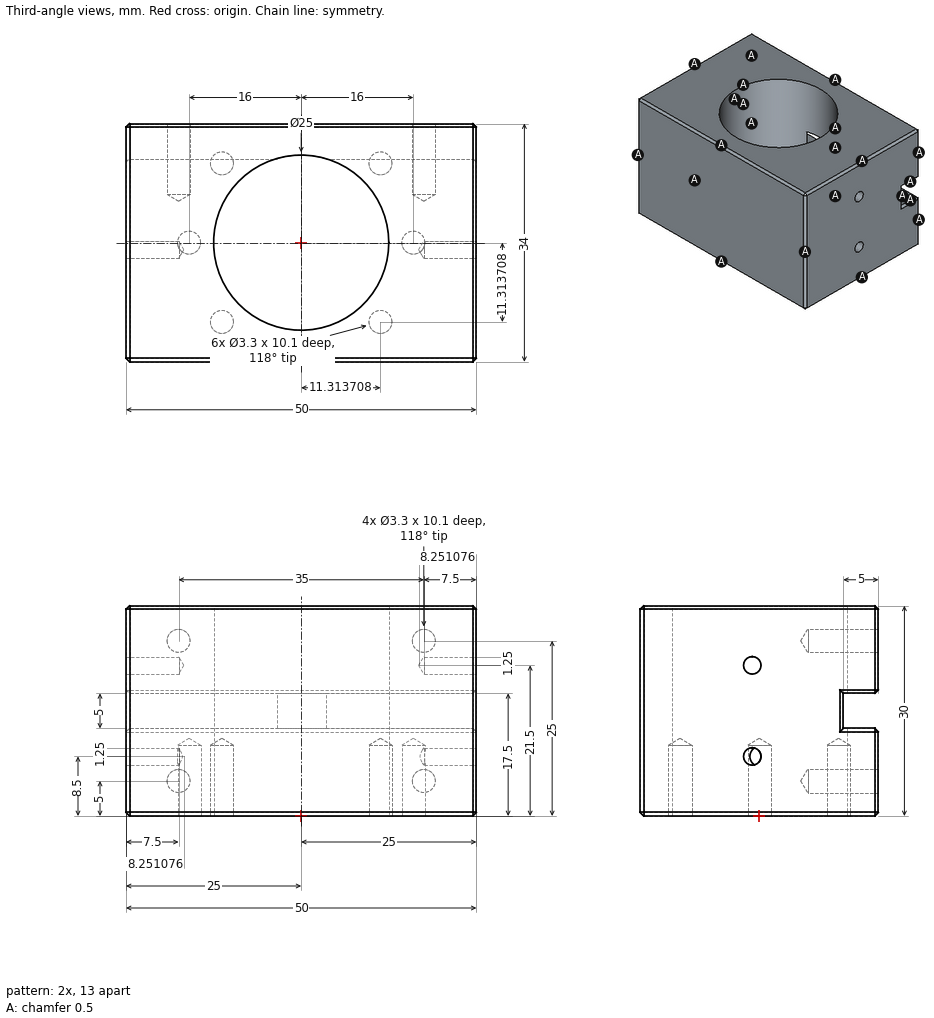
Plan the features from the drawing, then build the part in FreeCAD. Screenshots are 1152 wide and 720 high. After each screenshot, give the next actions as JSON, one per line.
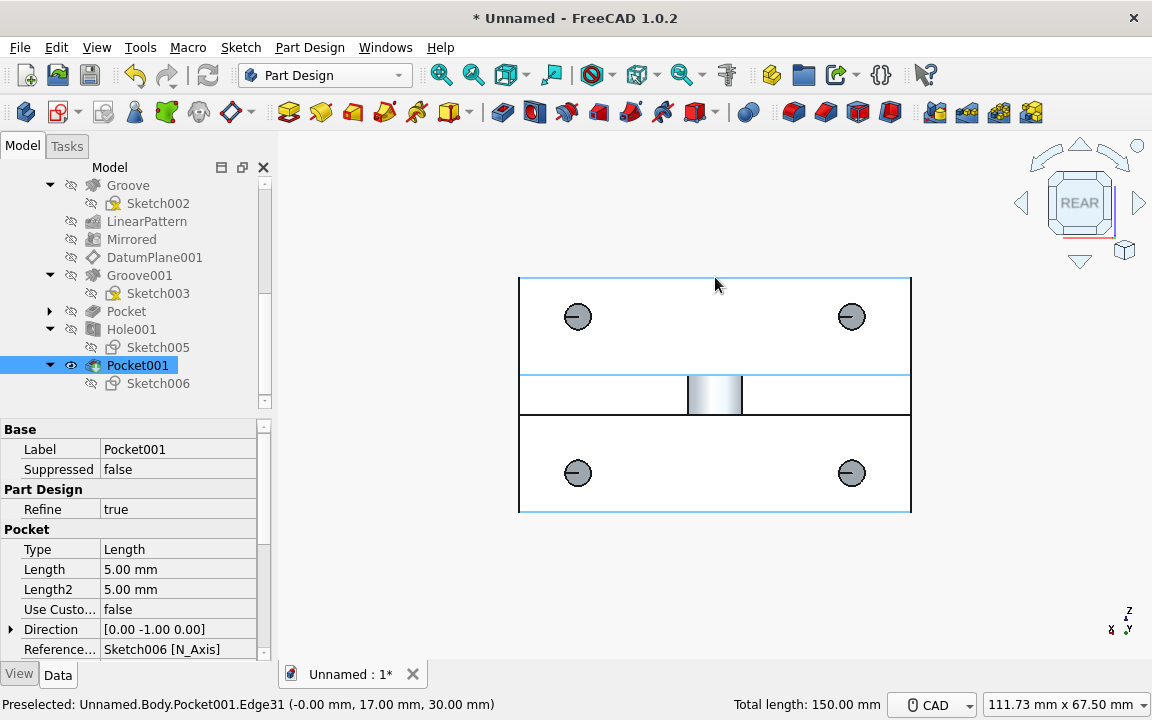
{"action": "left_click", "coordinate": [911, 326], "text": "ctrl"}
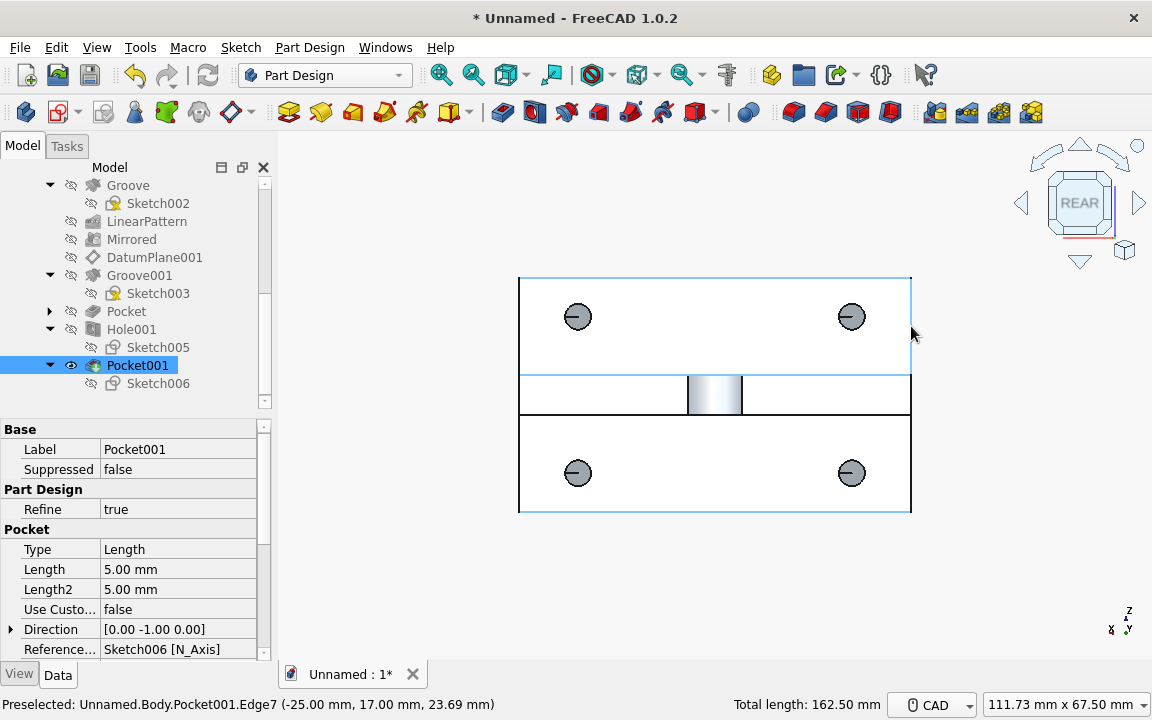
{"action": "left_click", "coordinate": [911, 462], "text": "ctrl"}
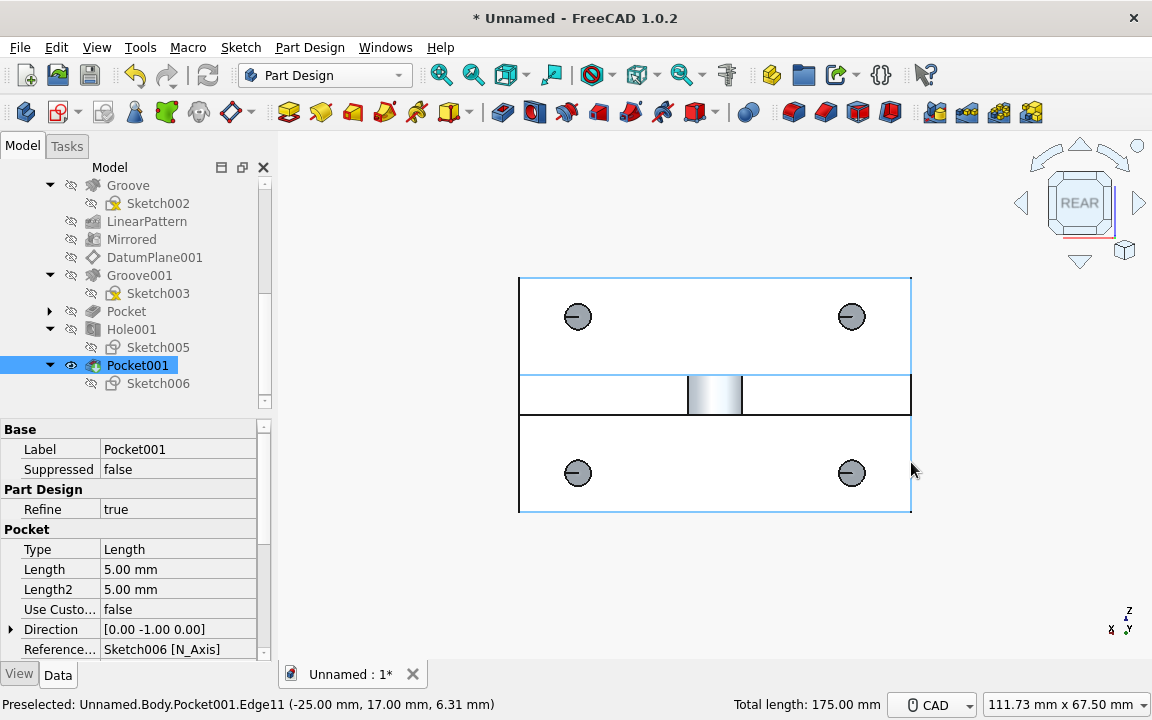
{"action": "left_click", "coordinate": [911, 394], "text": "ctrl"}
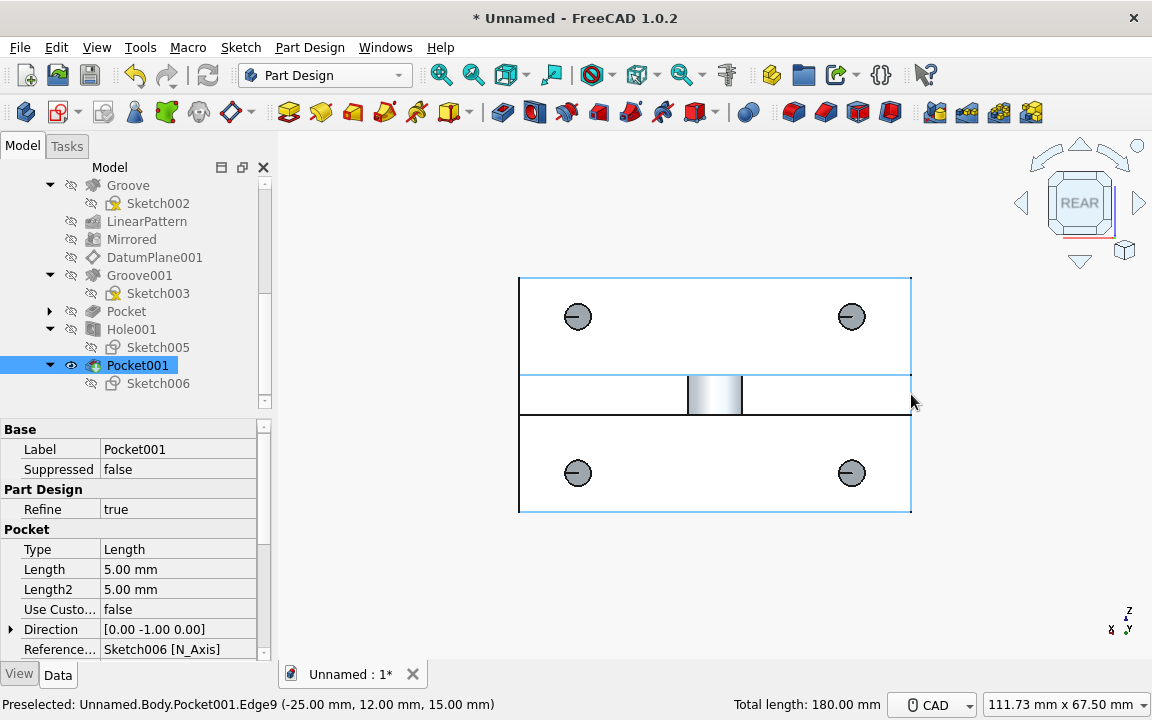
{"action": "left_click", "coordinate": [715, 414], "text": "ctrl"}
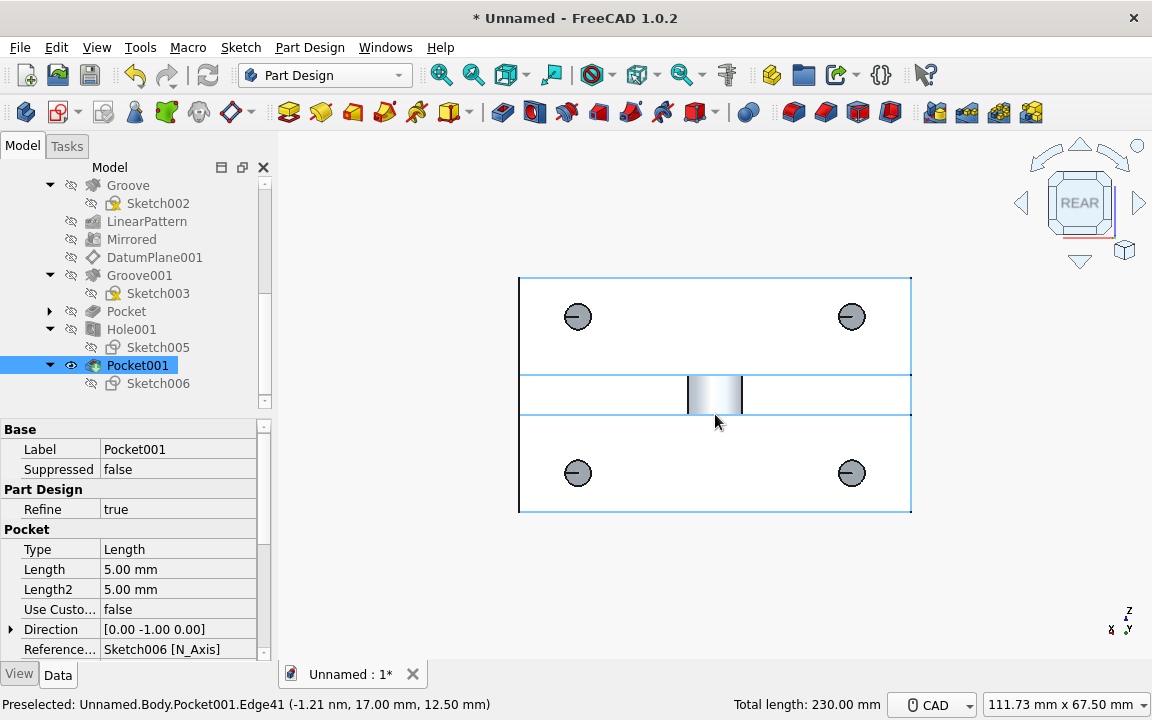
{"action": "key", "text": "0"}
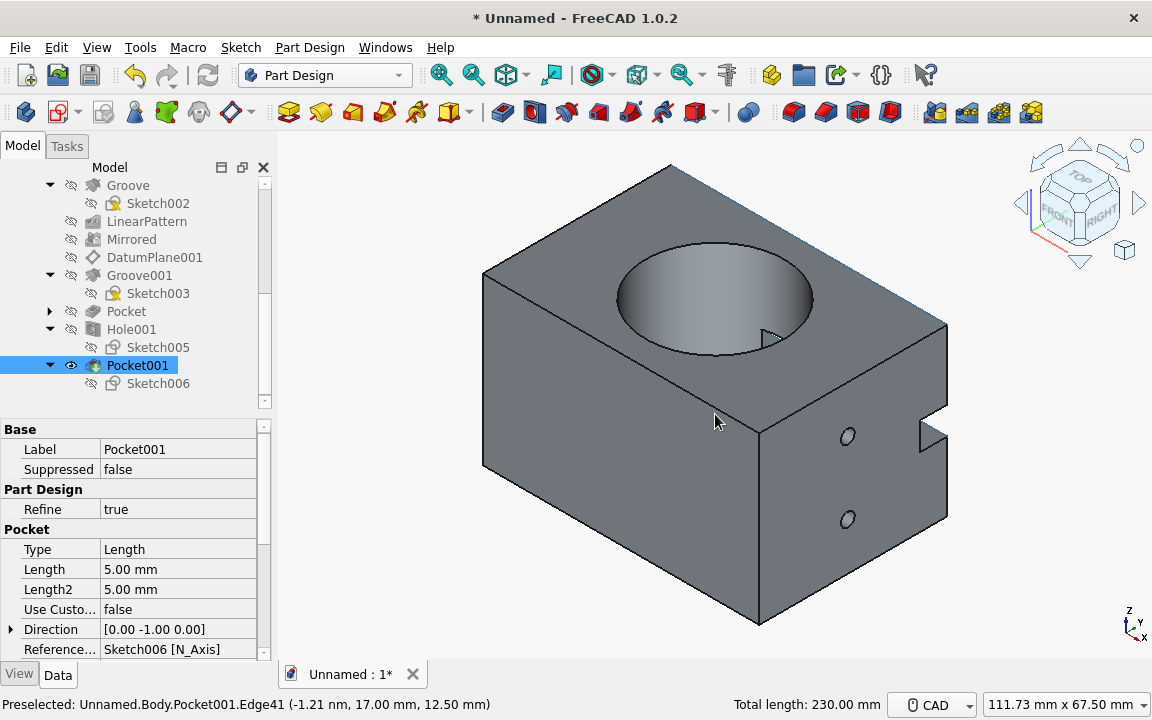
{"action": "left_click", "coordinate": [660, 471], "text": "ctrl"}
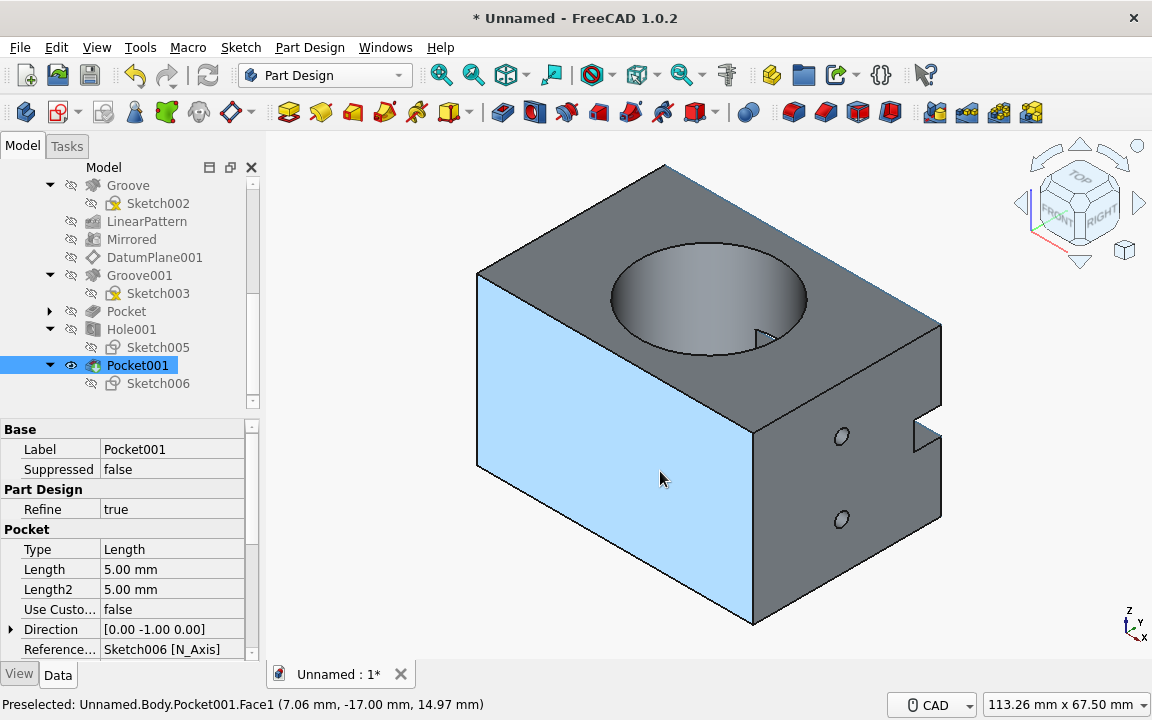
{"action": "left_click", "coordinate": [847, 378], "text": "ctrl"}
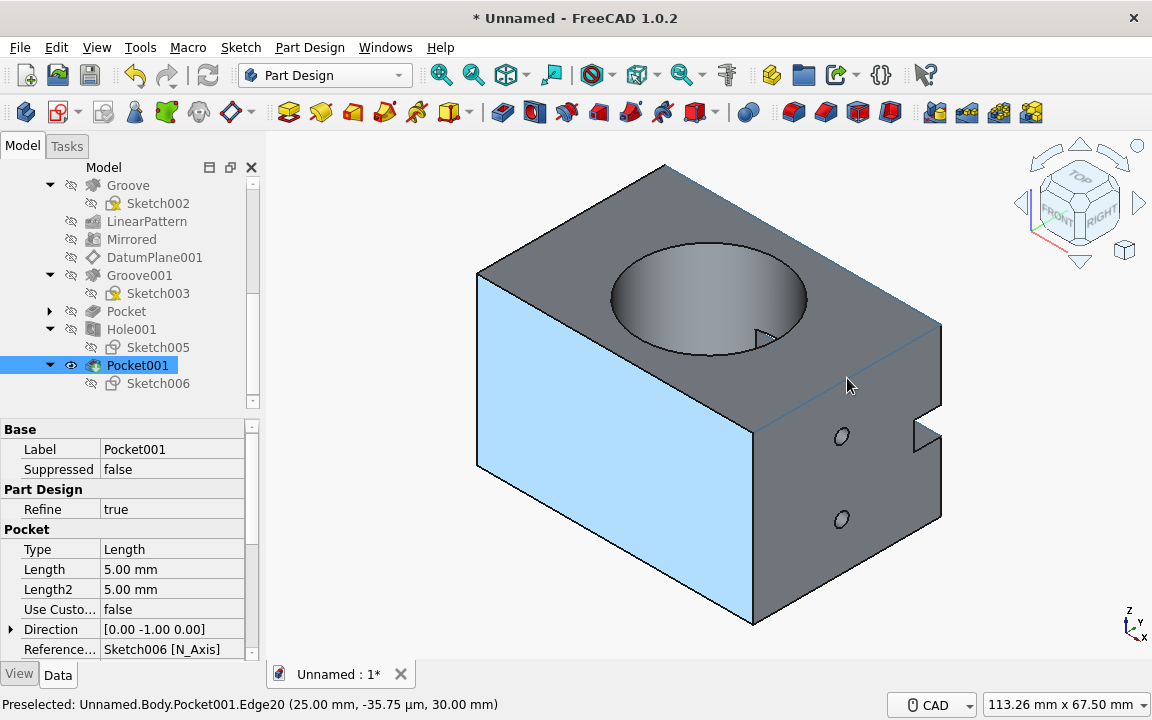
{"action": "left_click", "coordinate": [927, 443], "text": "ctrl"}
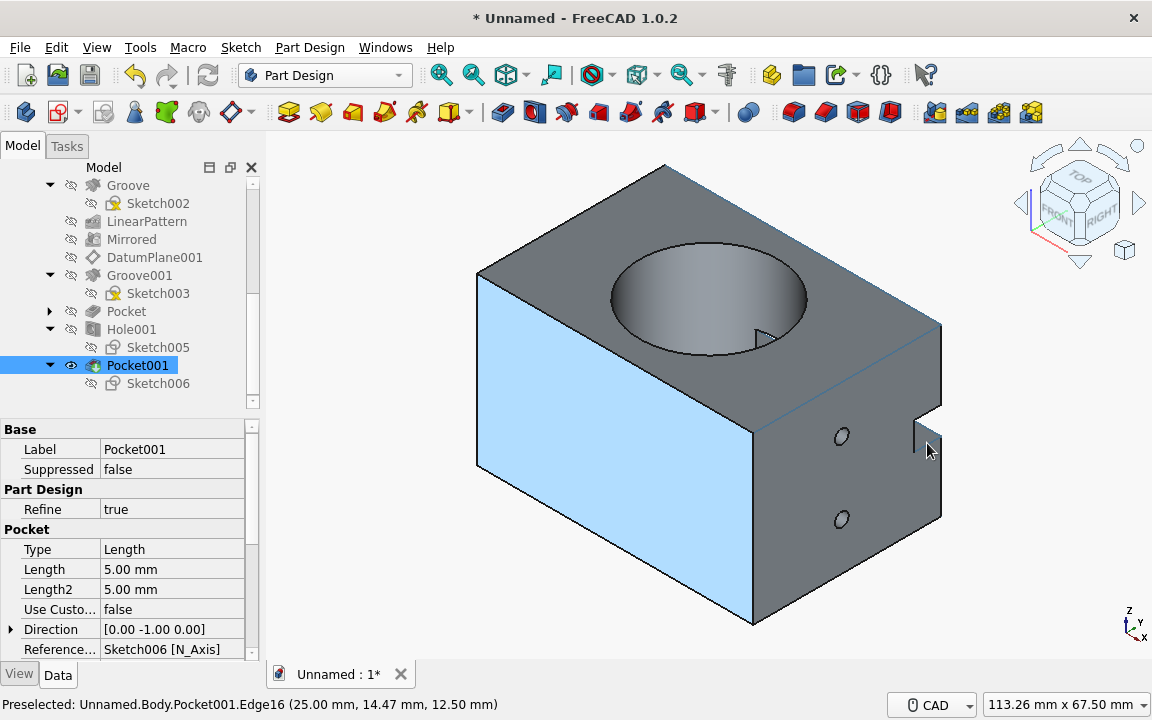
{"action": "key", "text": "2"}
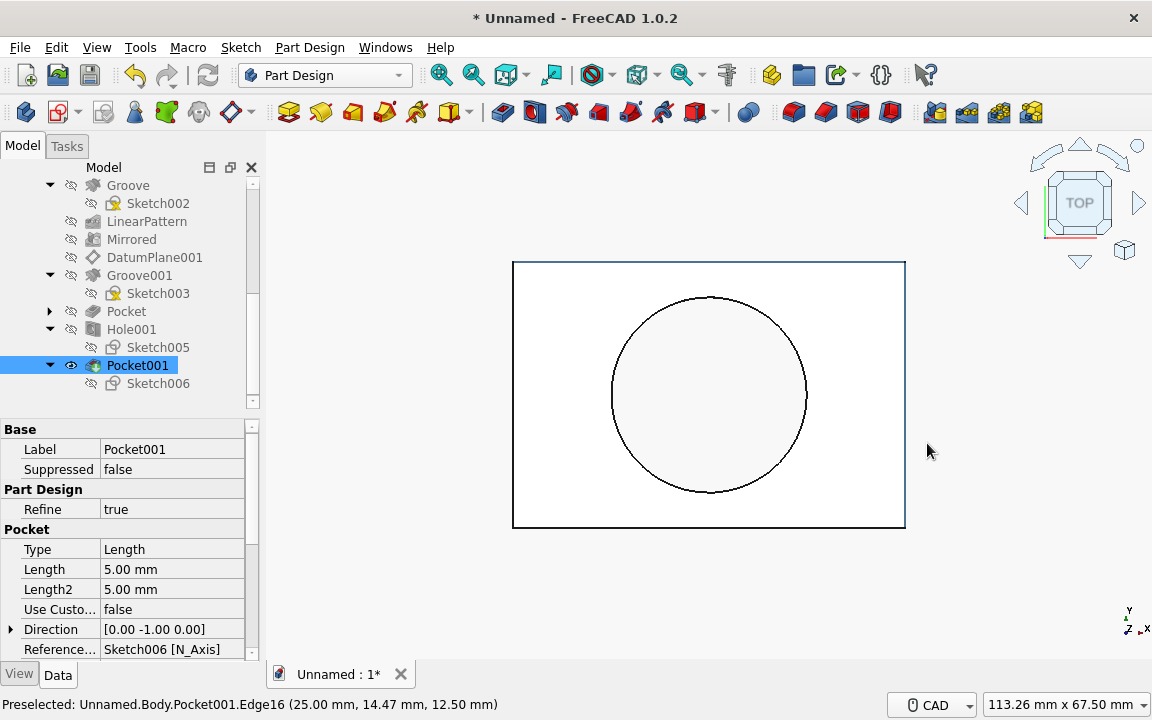
{"action": "left_click", "coordinate": [513, 394], "text": "ctrl"}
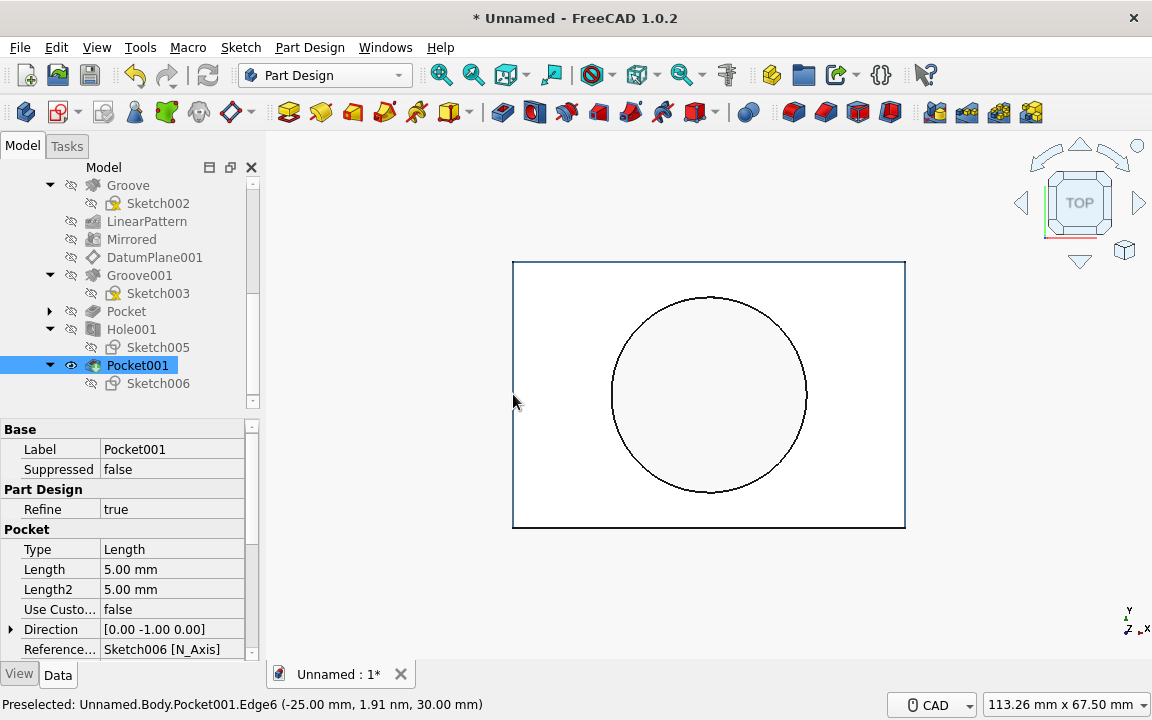
{"action": "key", "text": "1"}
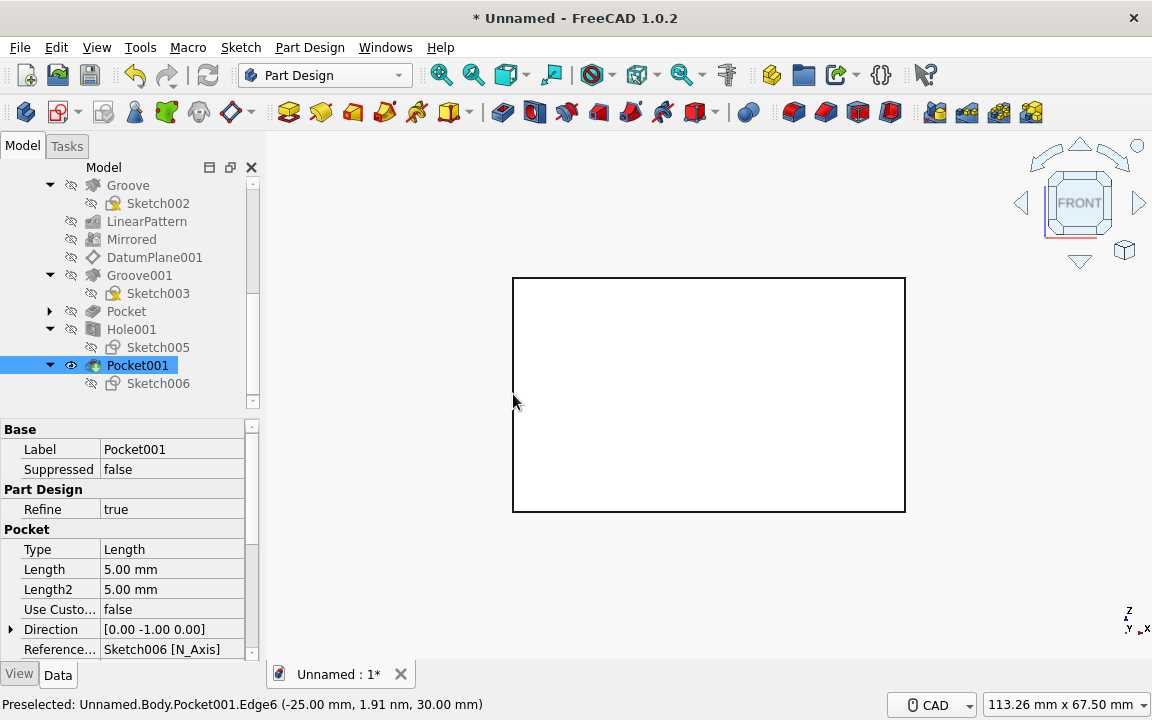
{"action": "key", "text": "v f"}